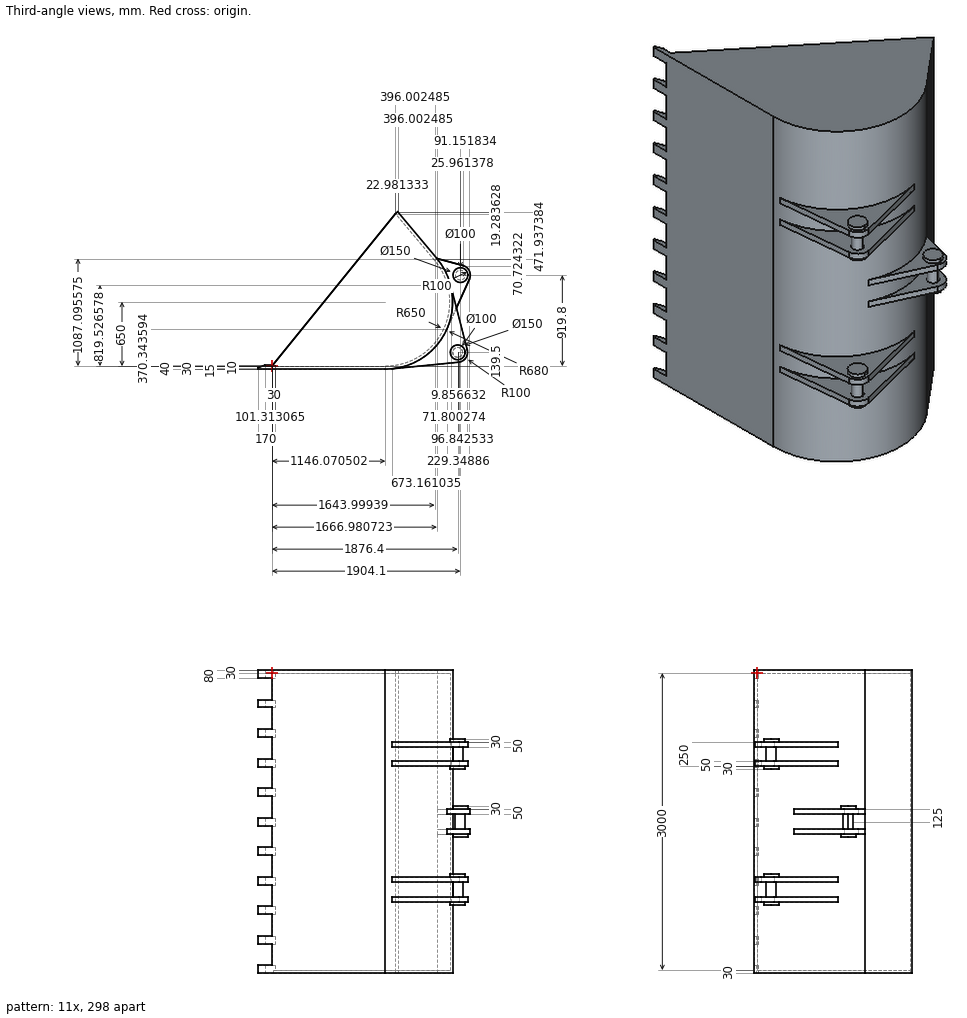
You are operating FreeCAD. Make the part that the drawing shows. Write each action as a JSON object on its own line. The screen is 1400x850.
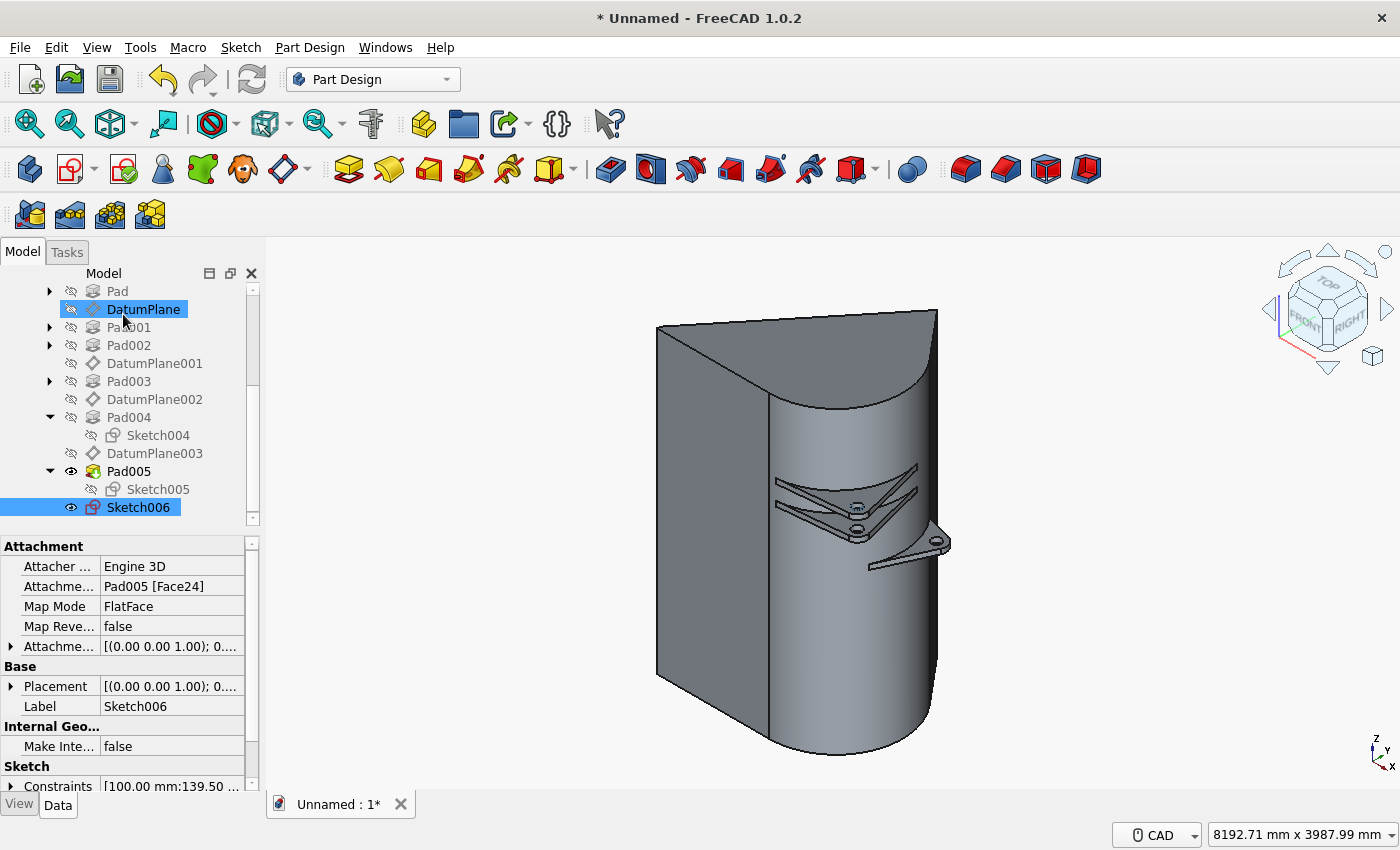
{"action": "left_click", "coordinate": [350, 170]}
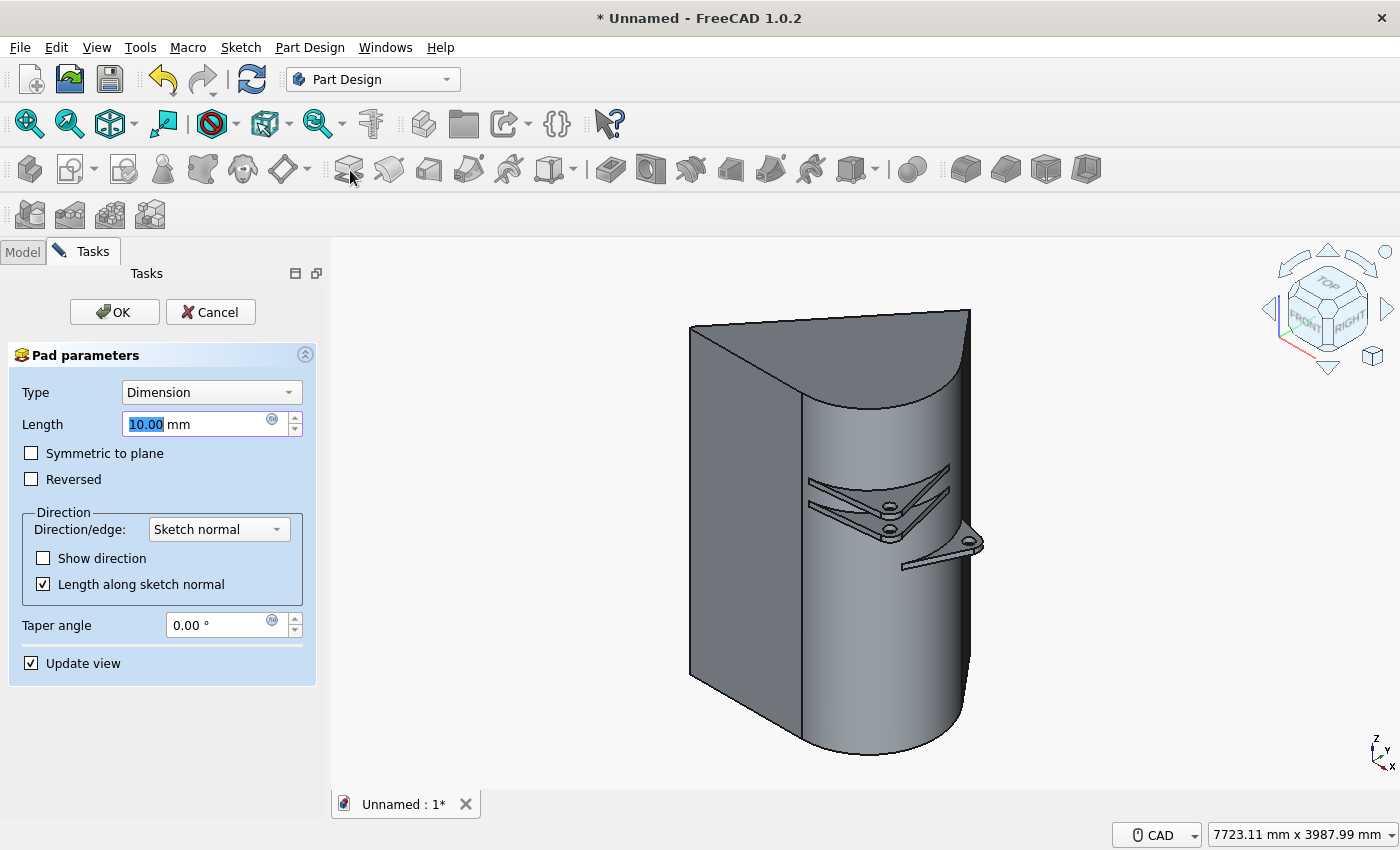
{"action": "type", "text": "250"}
{"action": "key", "text": "Tab"}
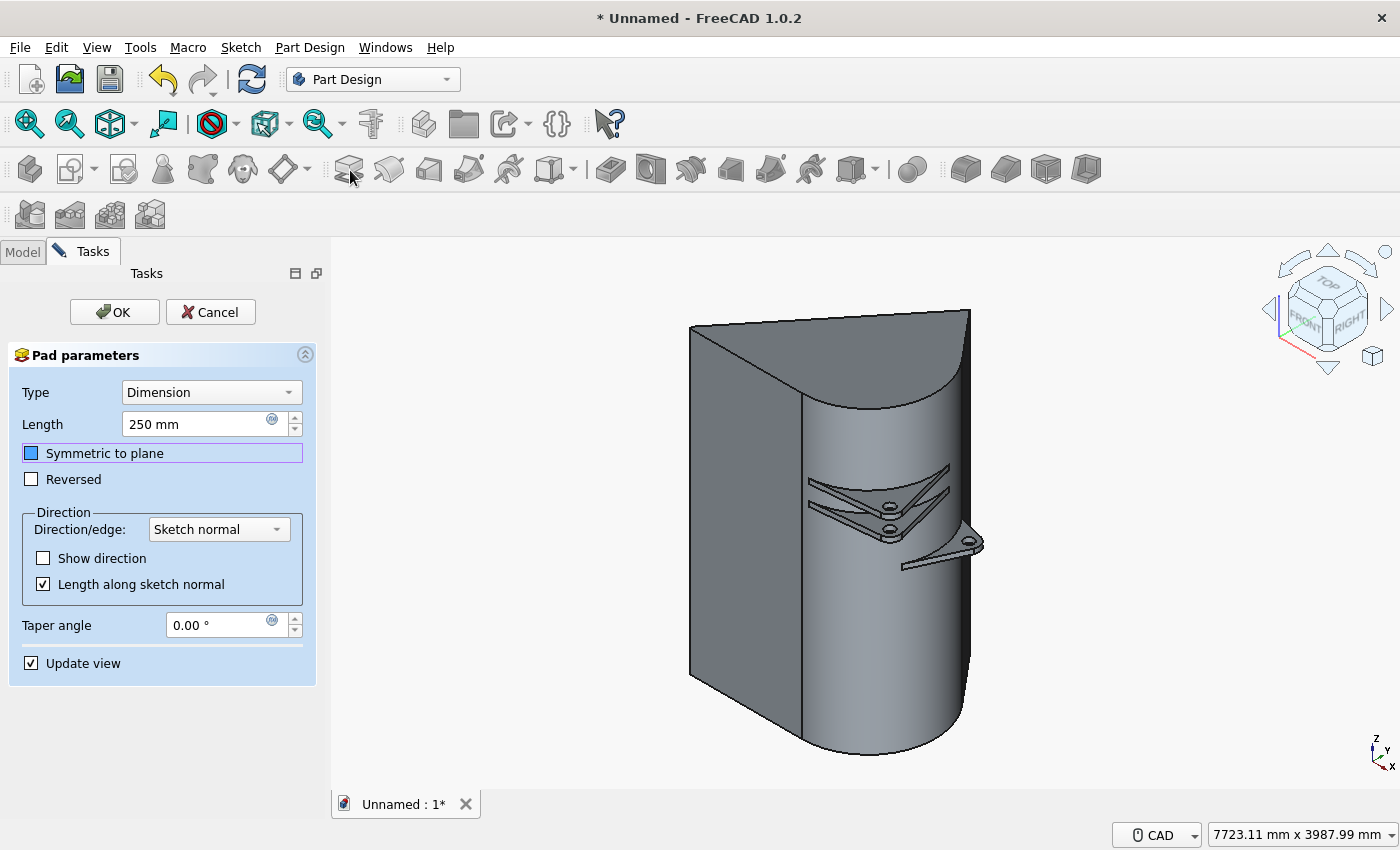
{"action": "left_click", "coordinate": [30, 479]}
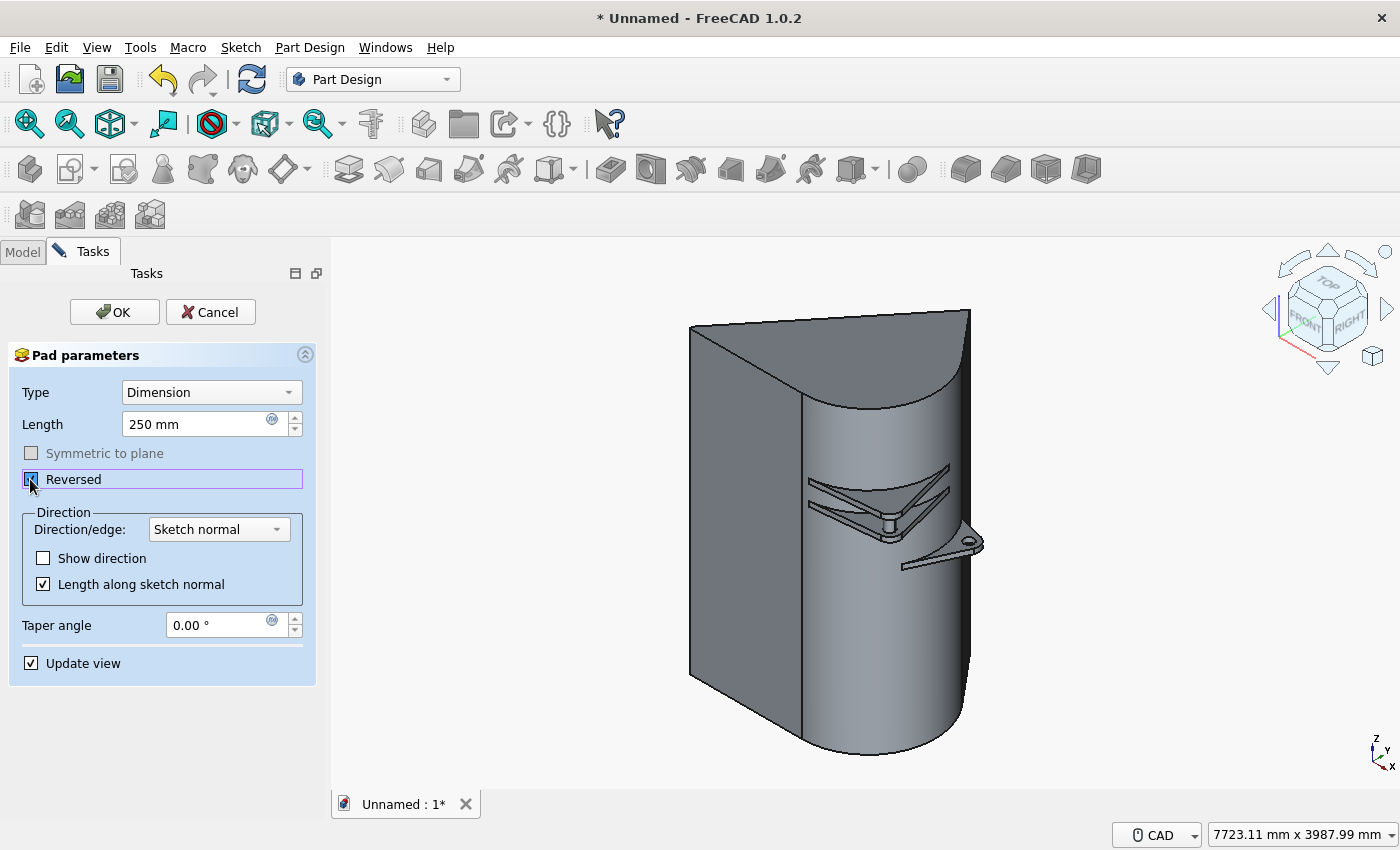
{"action": "left_click", "coordinate": [115, 312]}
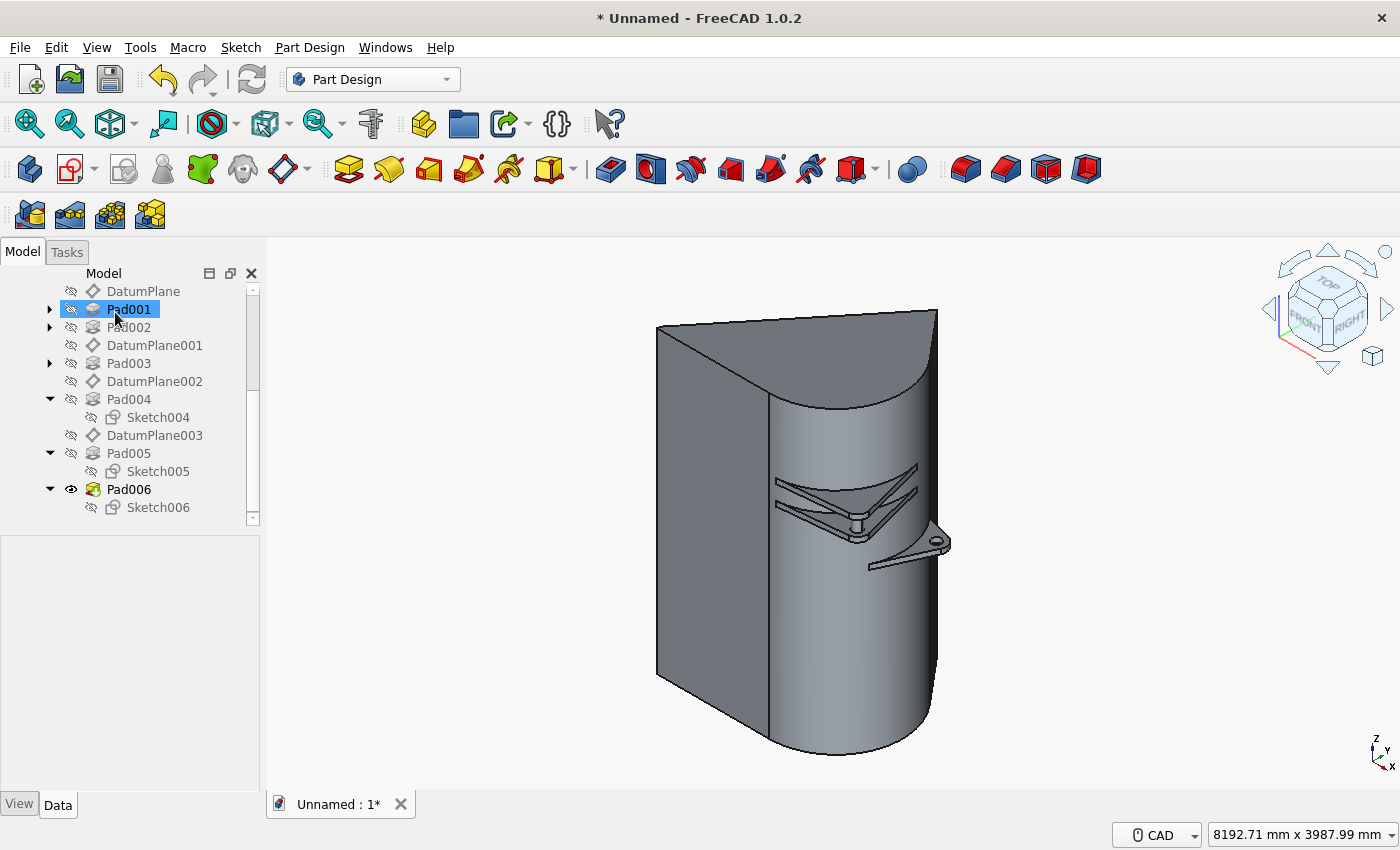
{"action": "scroll", "coordinate": [140, 395], "scroll_direction": "down", "scroll_amount": 3}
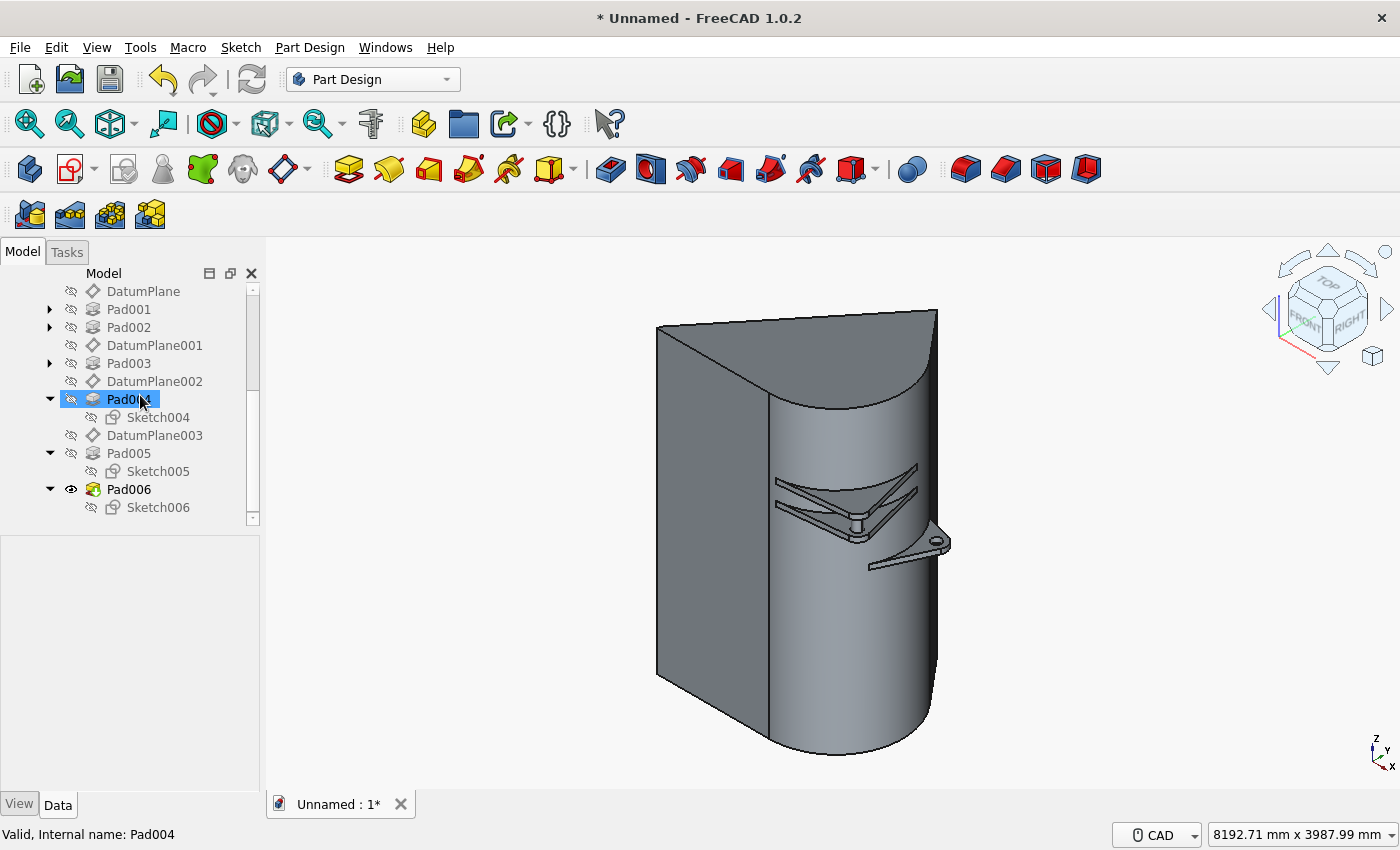
{"action": "scroll", "coordinate": [140, 395], "scroll_direction": "up", "scroll_amount": 15}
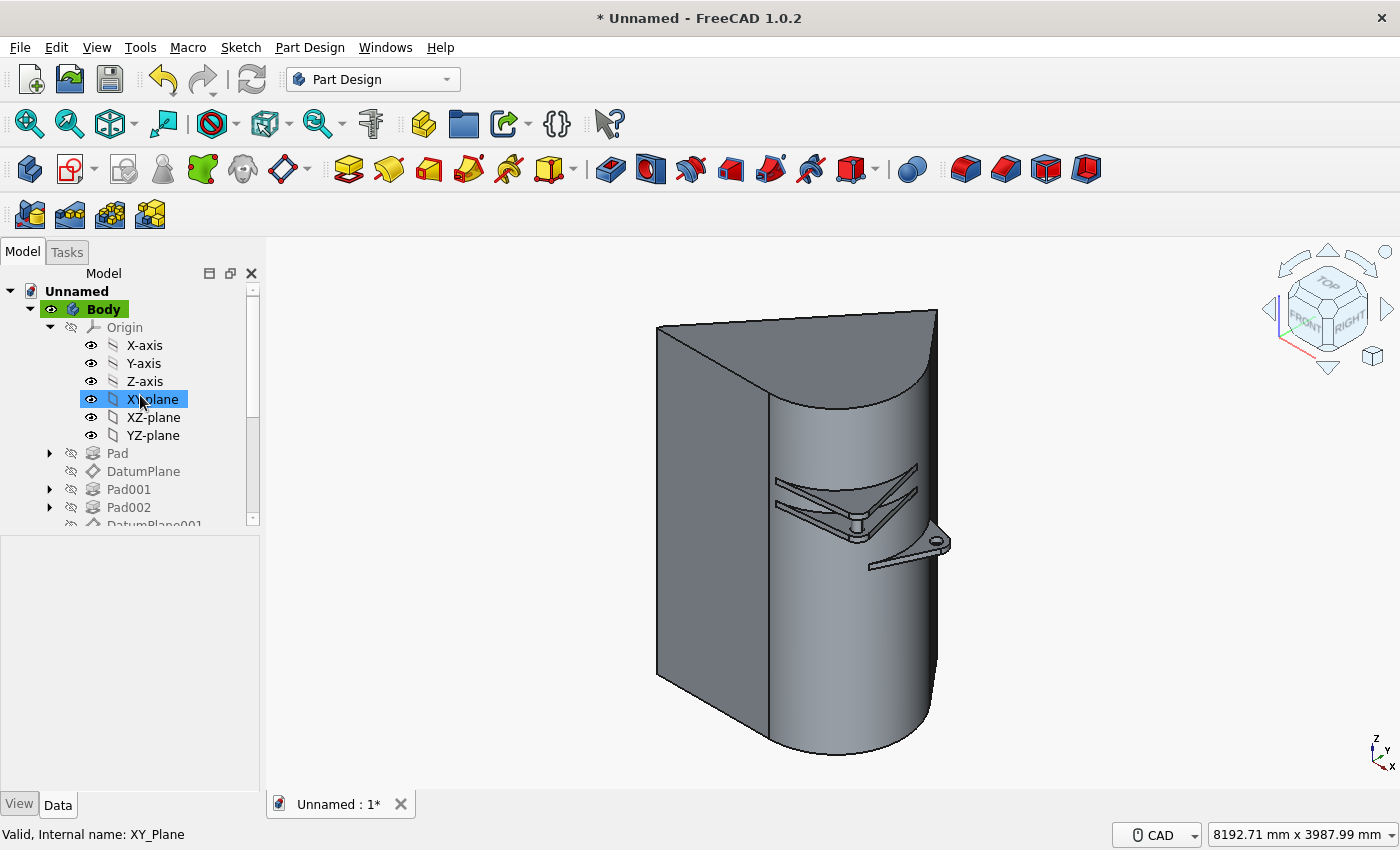
{"action": "left_click", "coordinate": [136, 399]}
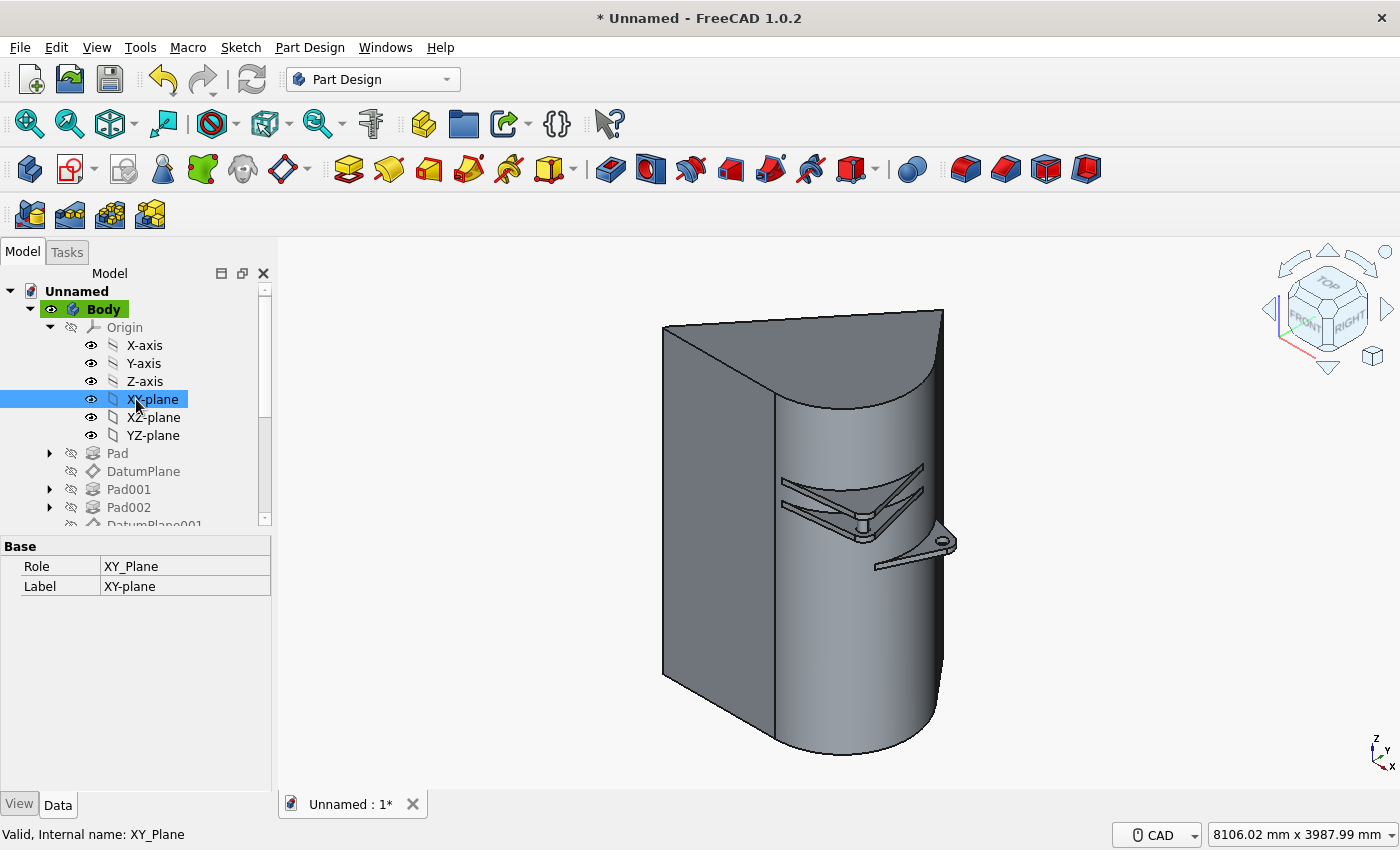
{"action": "left_click", "coordinate": [284, 170]}